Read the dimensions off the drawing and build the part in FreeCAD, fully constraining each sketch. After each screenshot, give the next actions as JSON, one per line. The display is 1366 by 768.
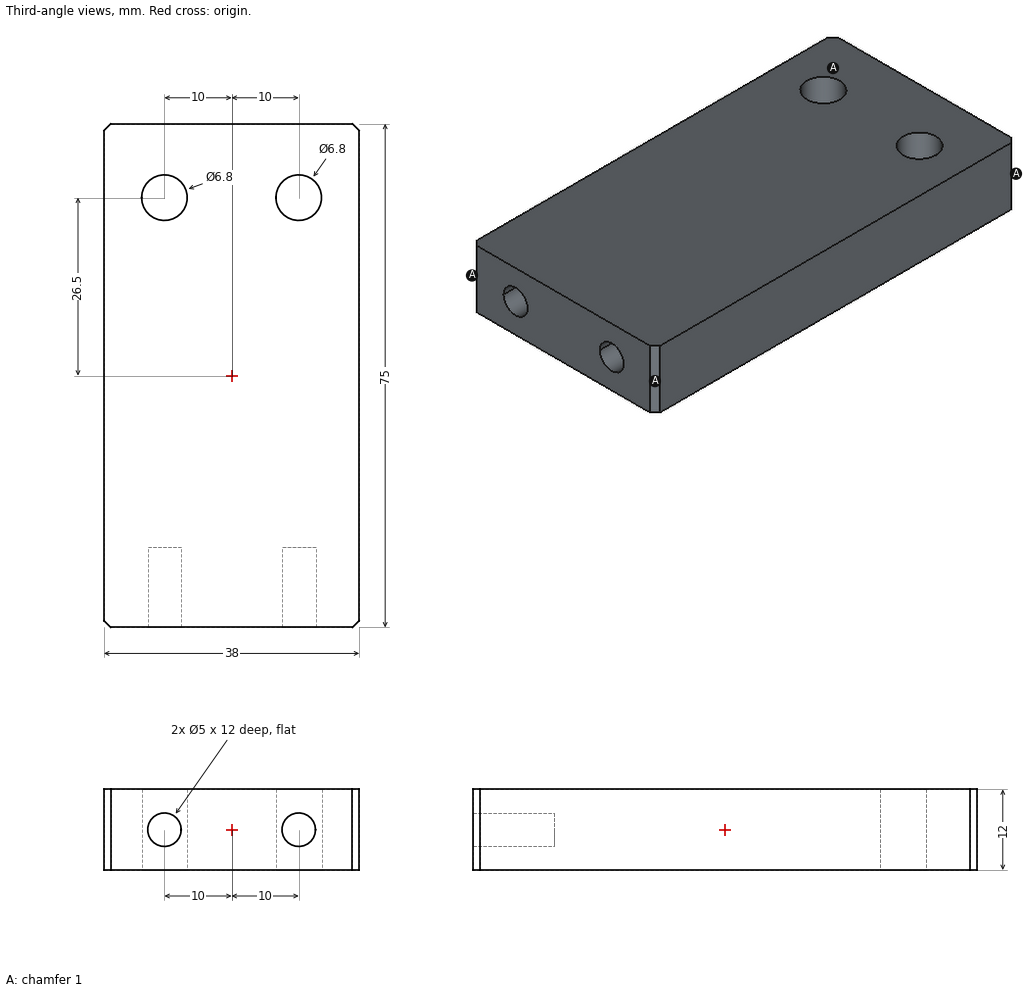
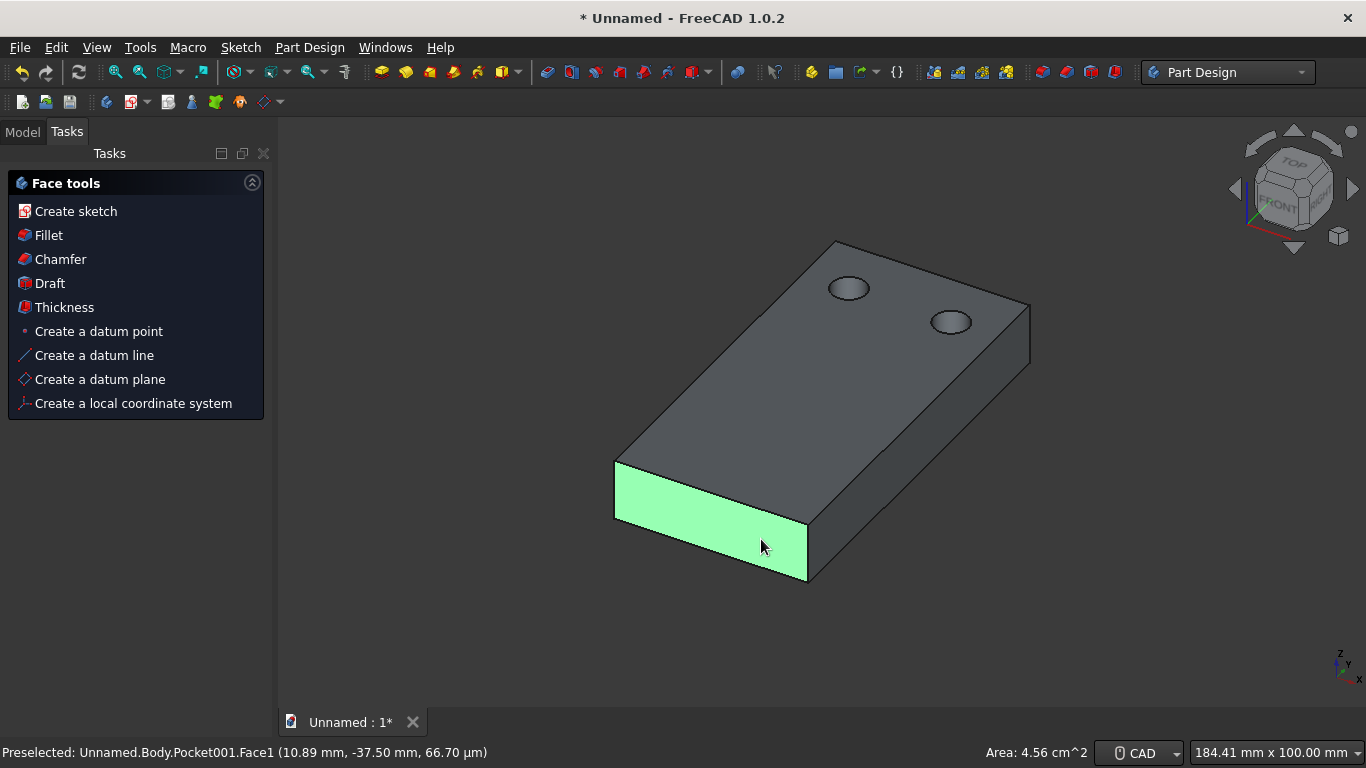
{"action": "left_click", "coordinate": [132, 102]}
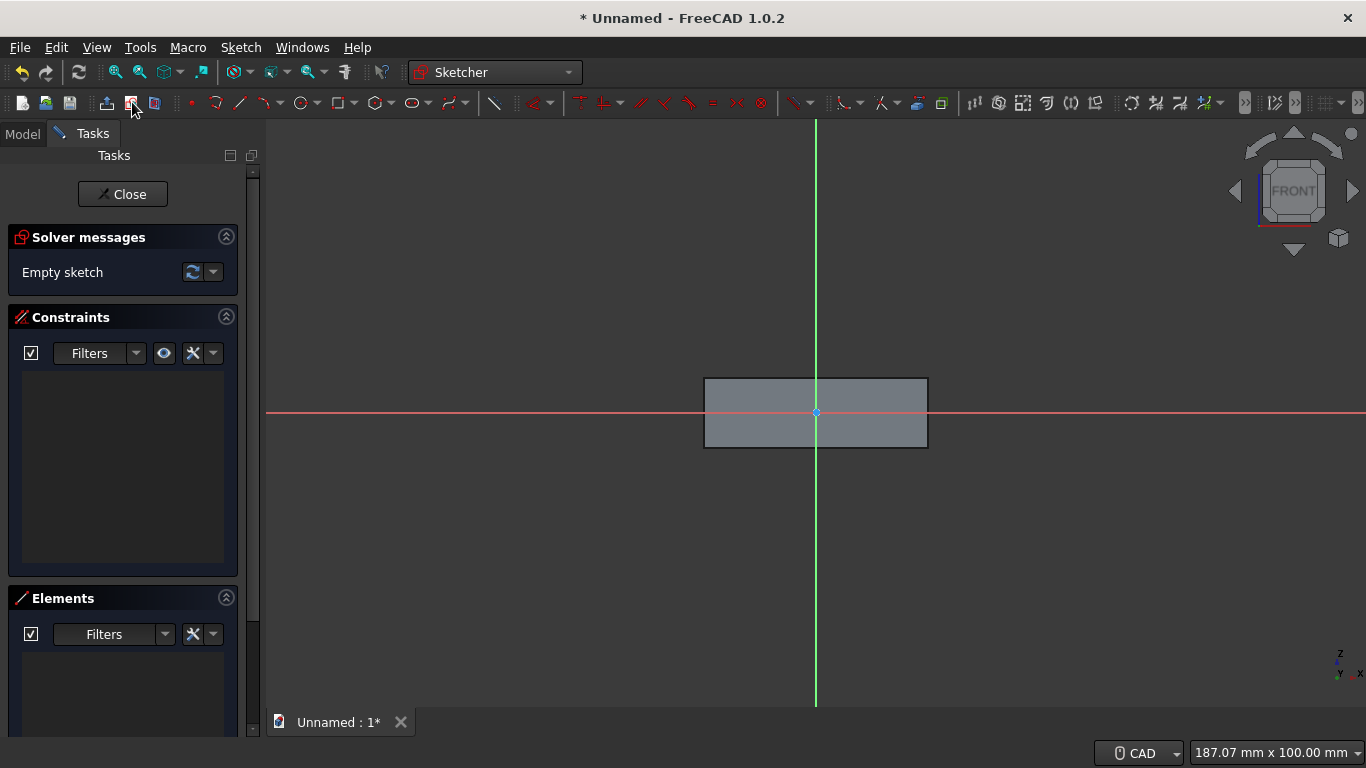
{"action": "scroll", "coordinate": [838, 413], "scroll_direction": "up", "scroll_amount": 7}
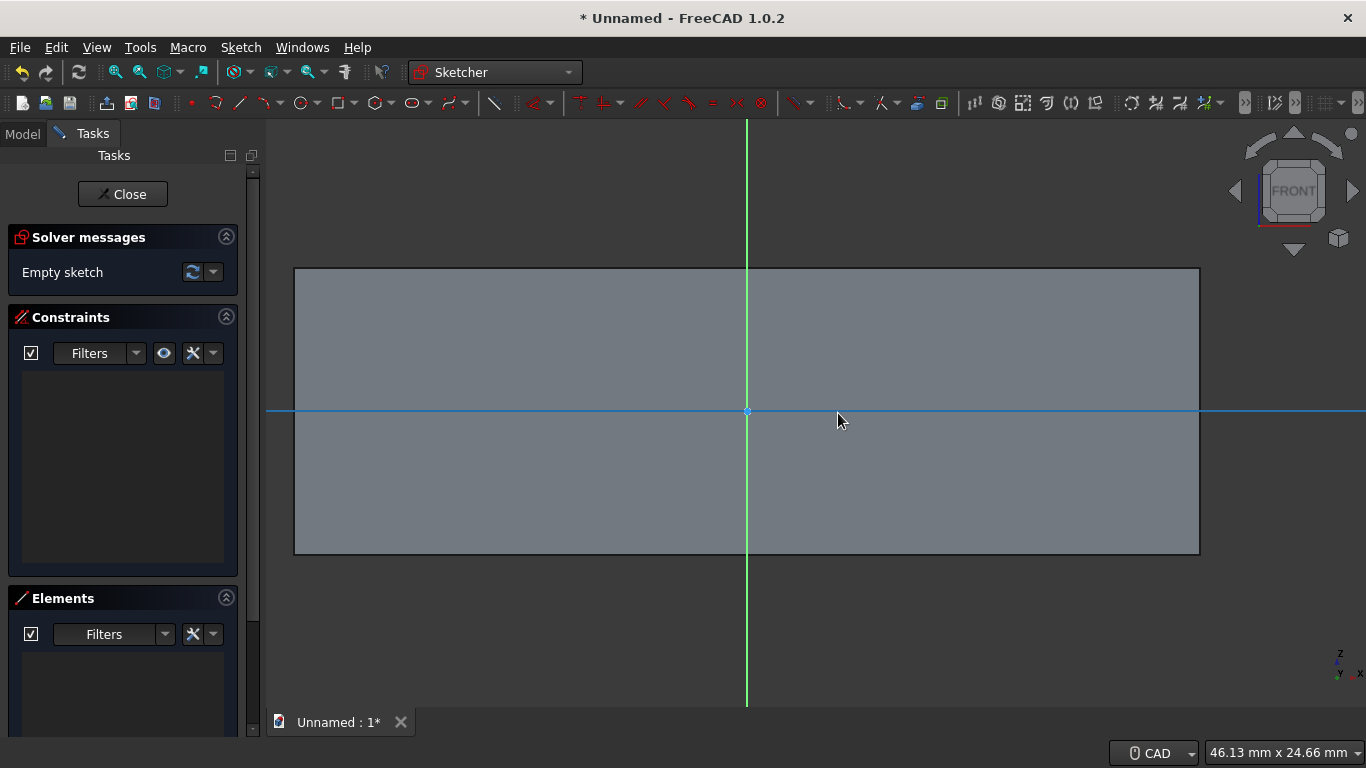
{"action": "key", "text": "g c"}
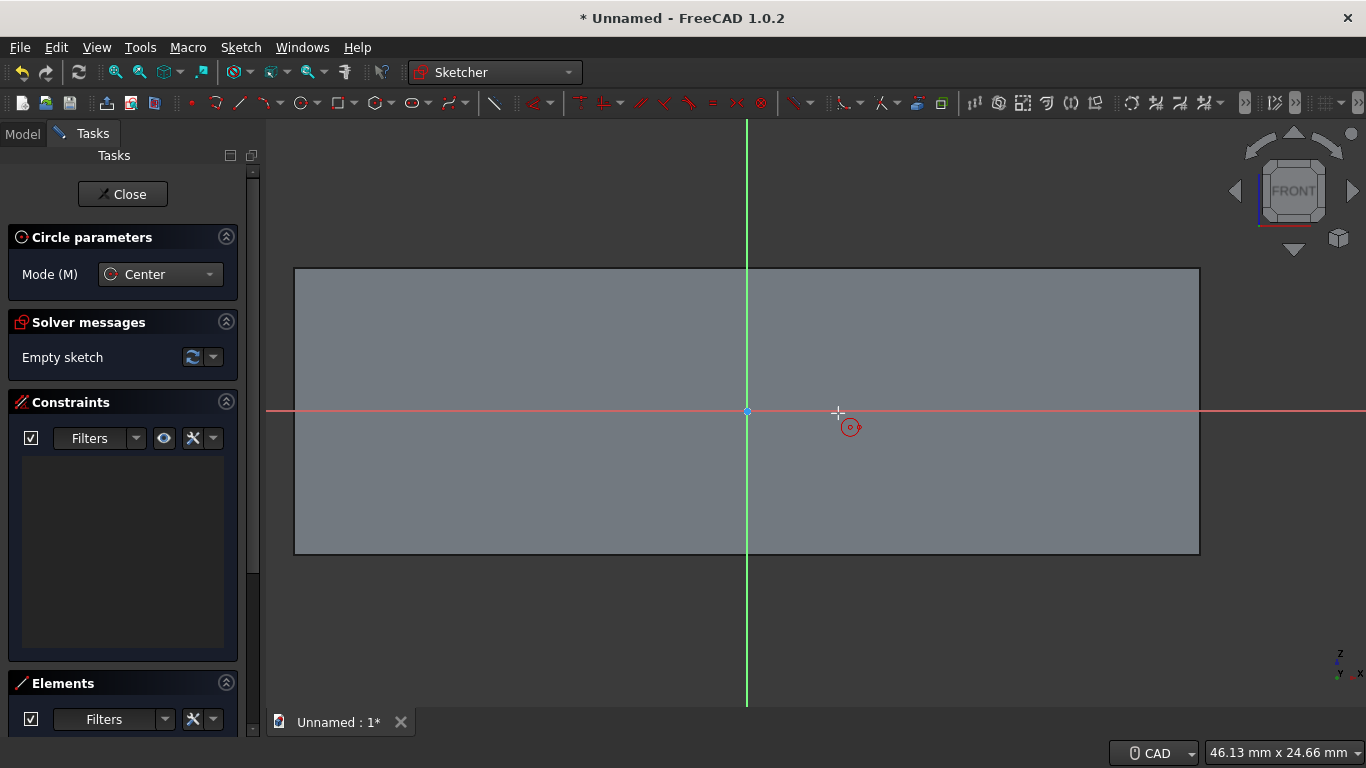
{"action": "left_click", "coordinate": [509, 411]}
{"action": "mouse_move", "coordinate": [551, 369]}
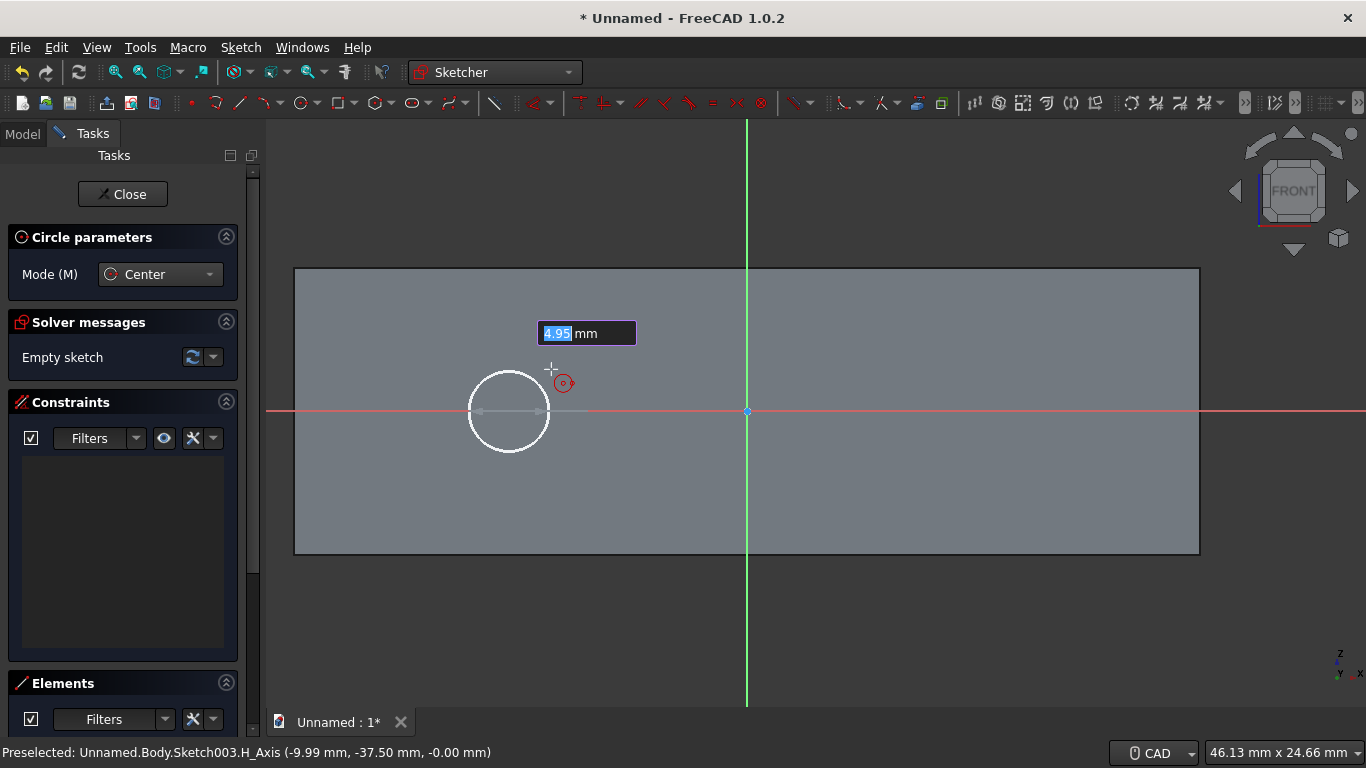
{"action": "type", "text": "5"}
{"action": "key", "text": "Return"}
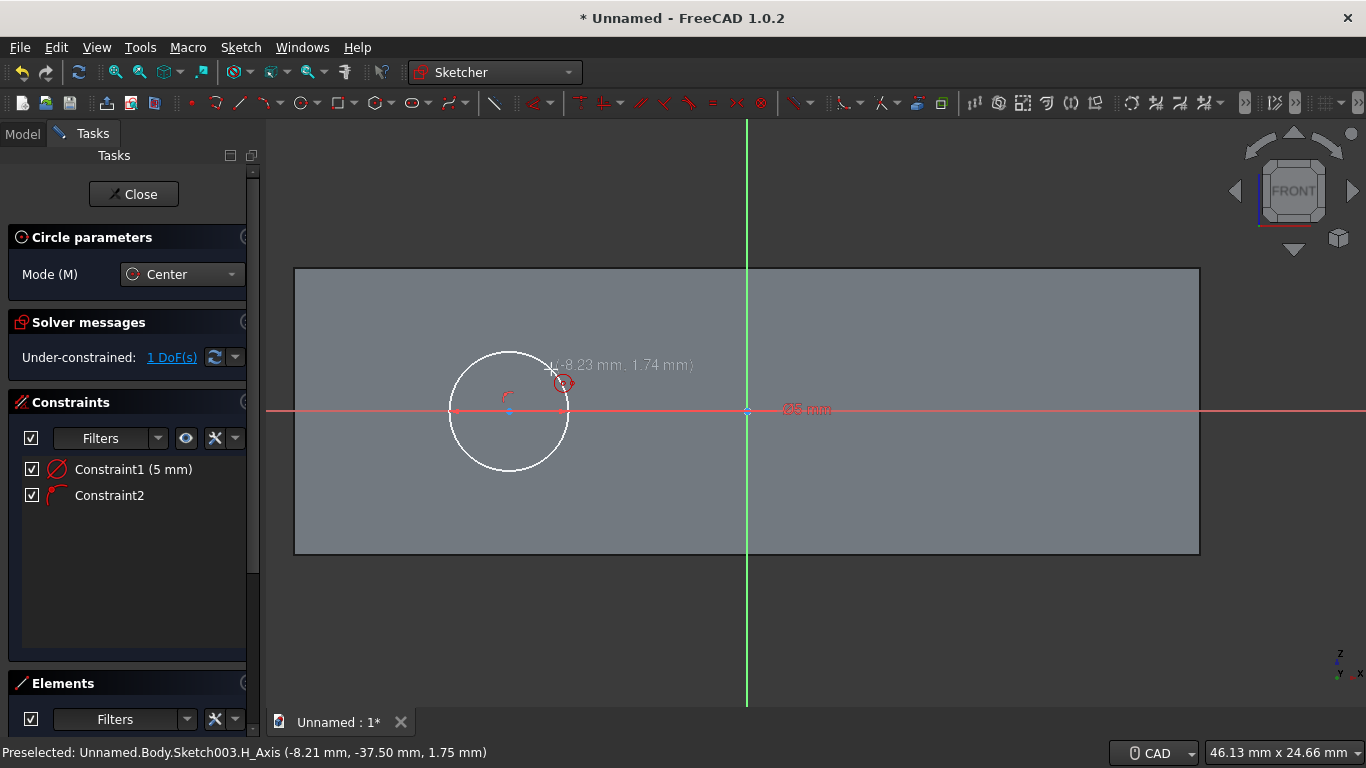
{"action": "left_click", "coordinate": [986, 411]}
{"action": "mouse_move", "coordinate": [1028, 369]}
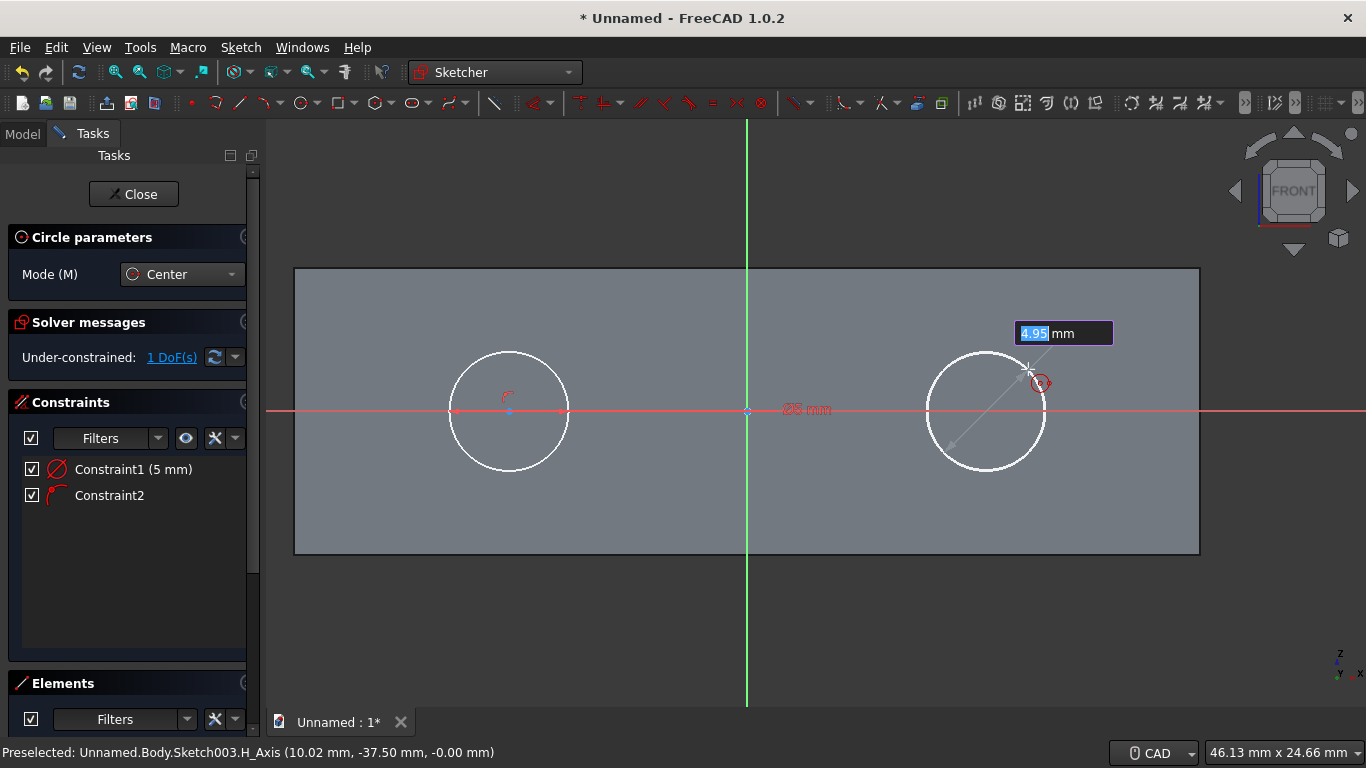
{"action": "type", "text": "5"}
{"action": "key", "text": "Return"}
{"action": "key", "text": "Escape"}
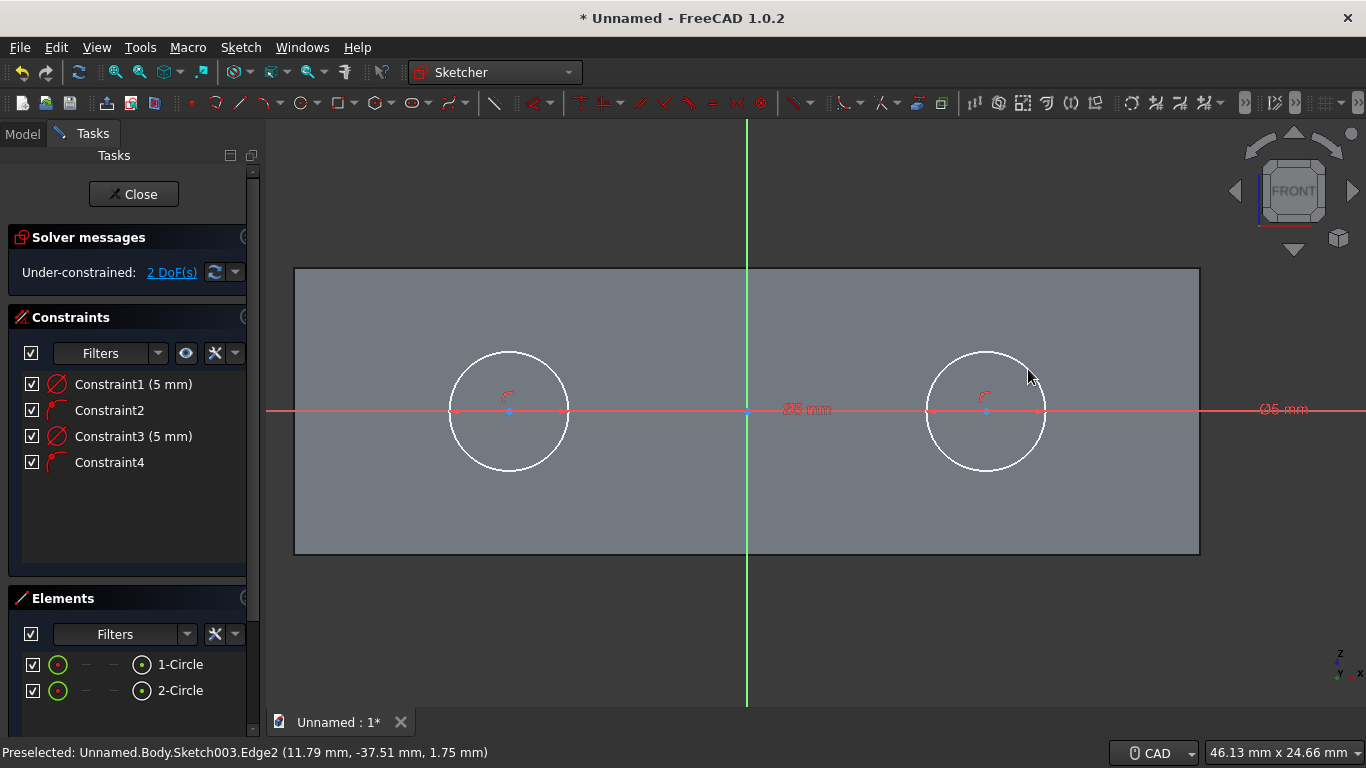
{"action": "key", "text": "d"}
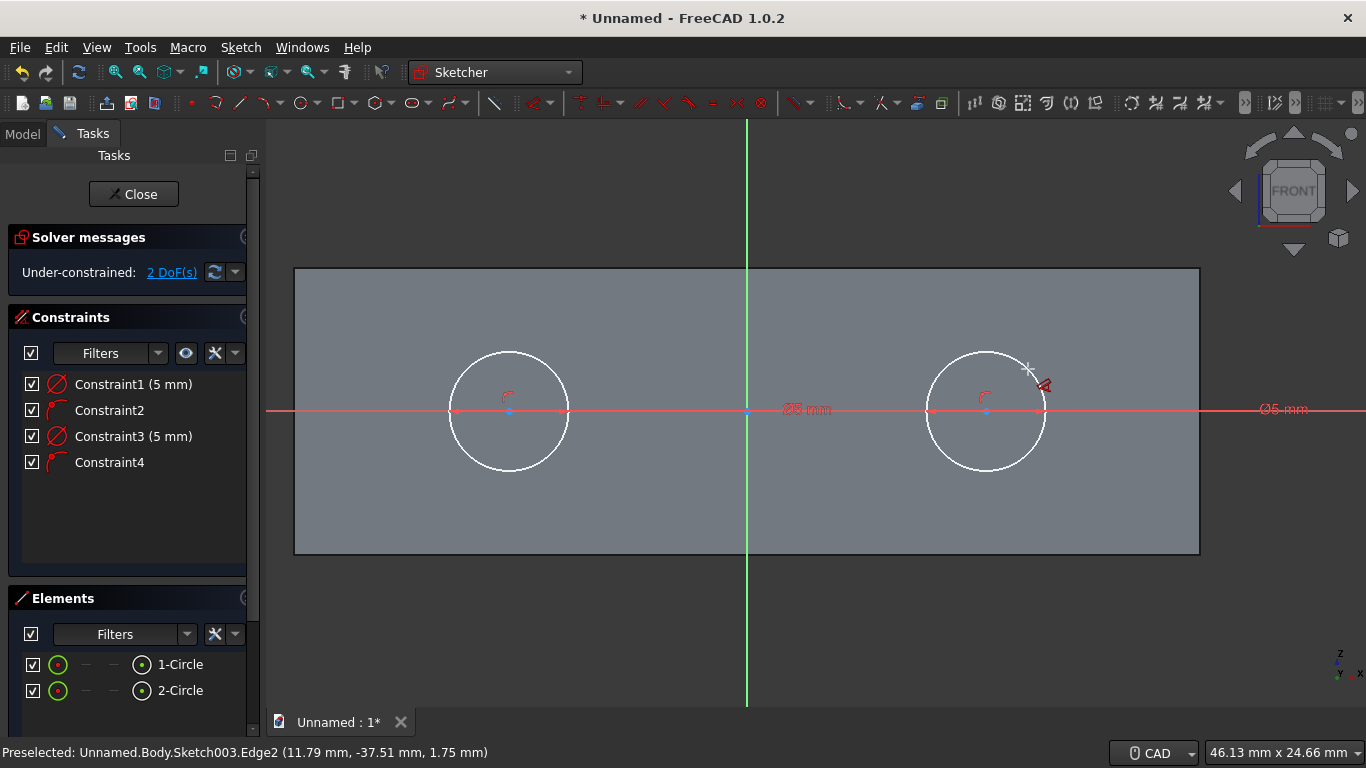
{"action": "left_click", "coordinate": [509, 411]}
{"action": "left_click", "coordinate": [628, 445]}